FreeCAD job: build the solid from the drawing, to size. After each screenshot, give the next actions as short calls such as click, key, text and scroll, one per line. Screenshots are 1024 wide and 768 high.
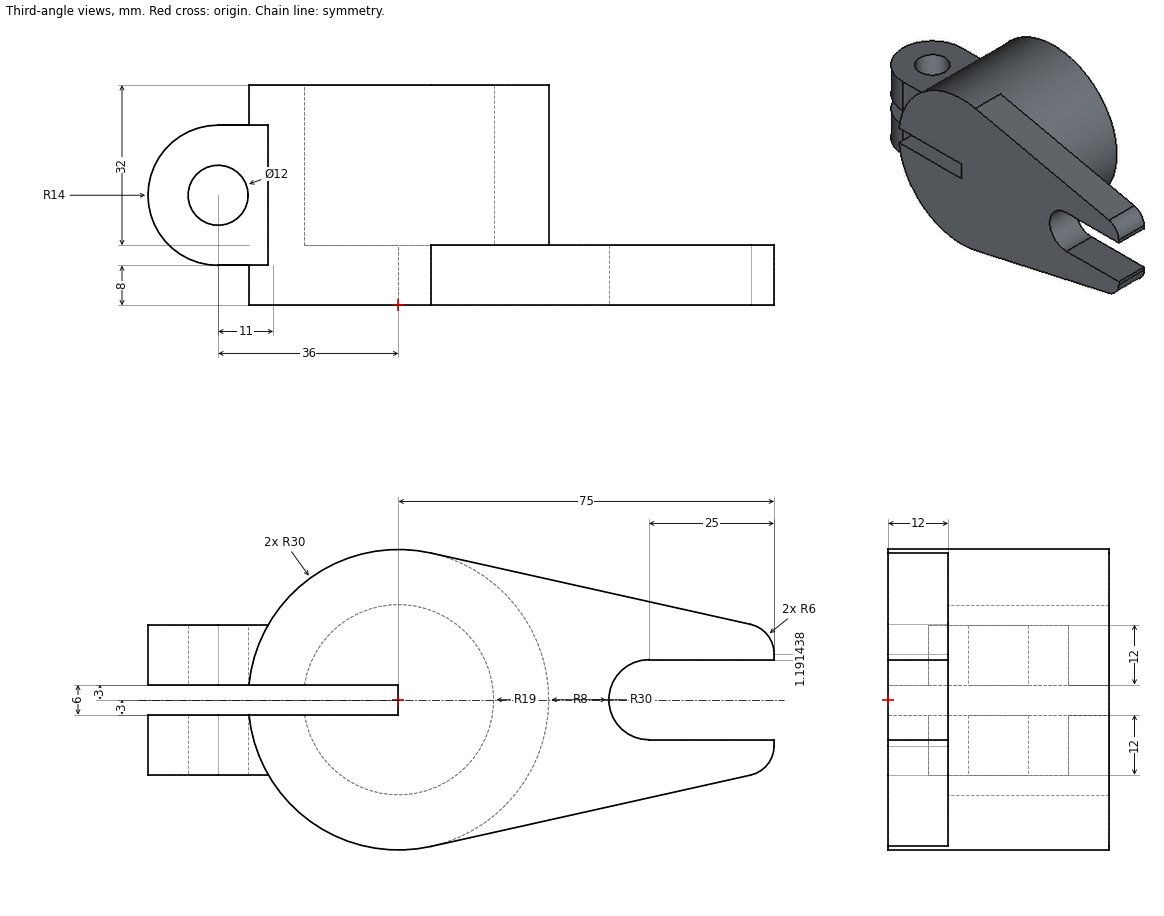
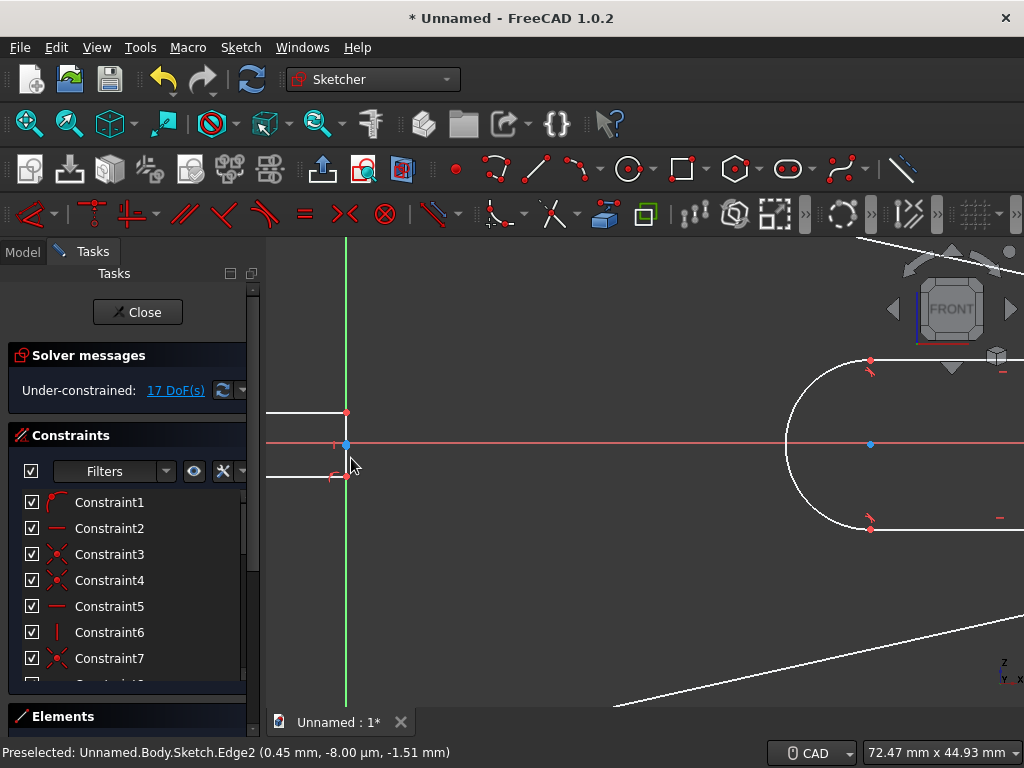
scroll(573, 489, down, 5)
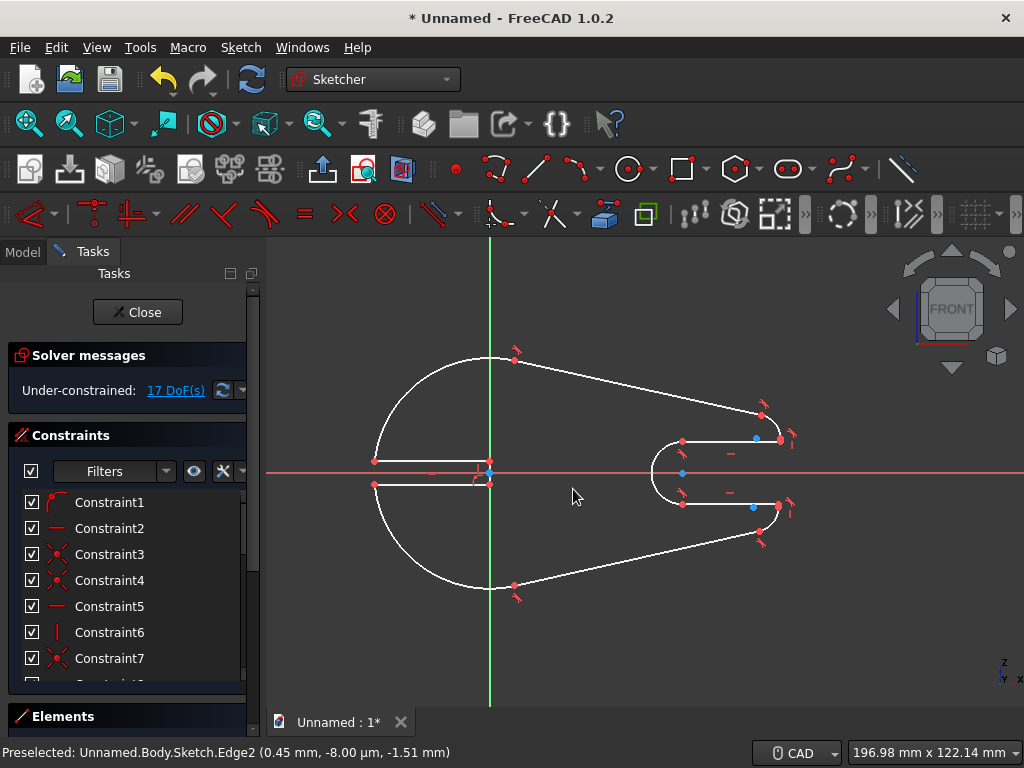
click(457, 363)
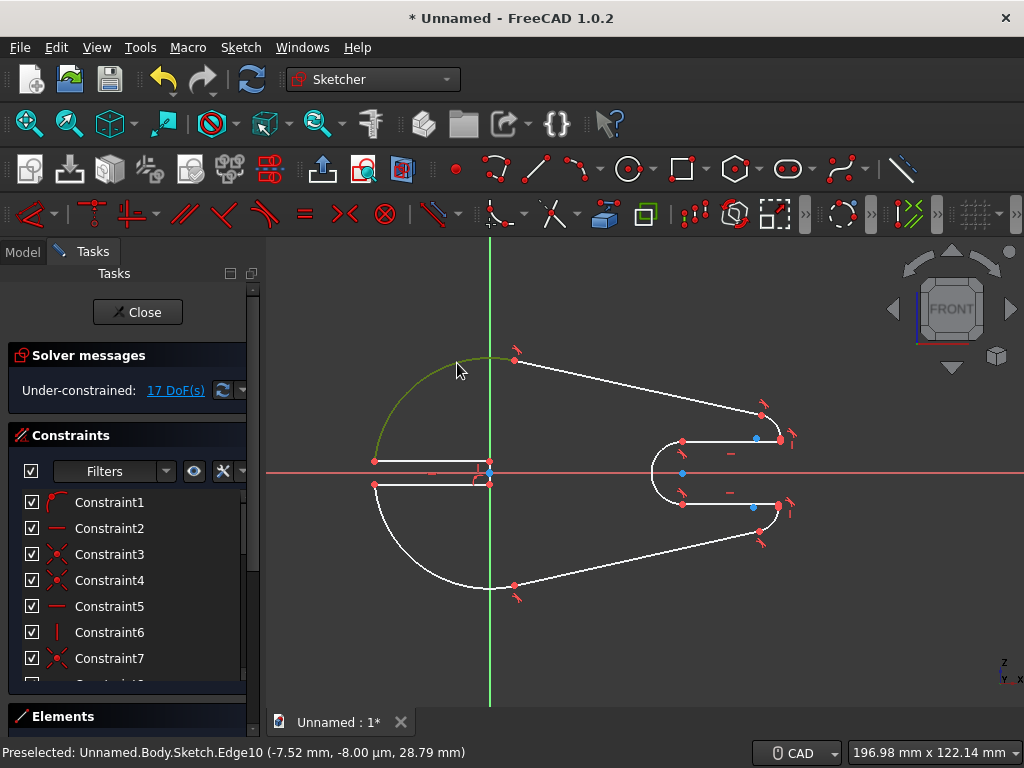
click(395, 539)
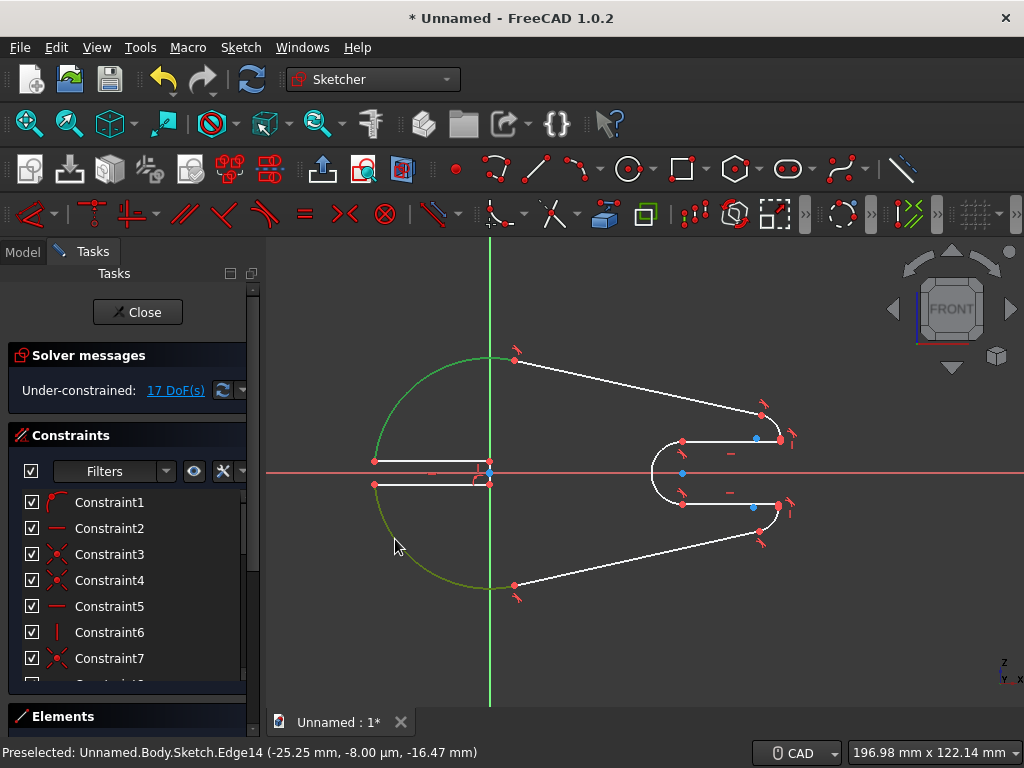
key(c)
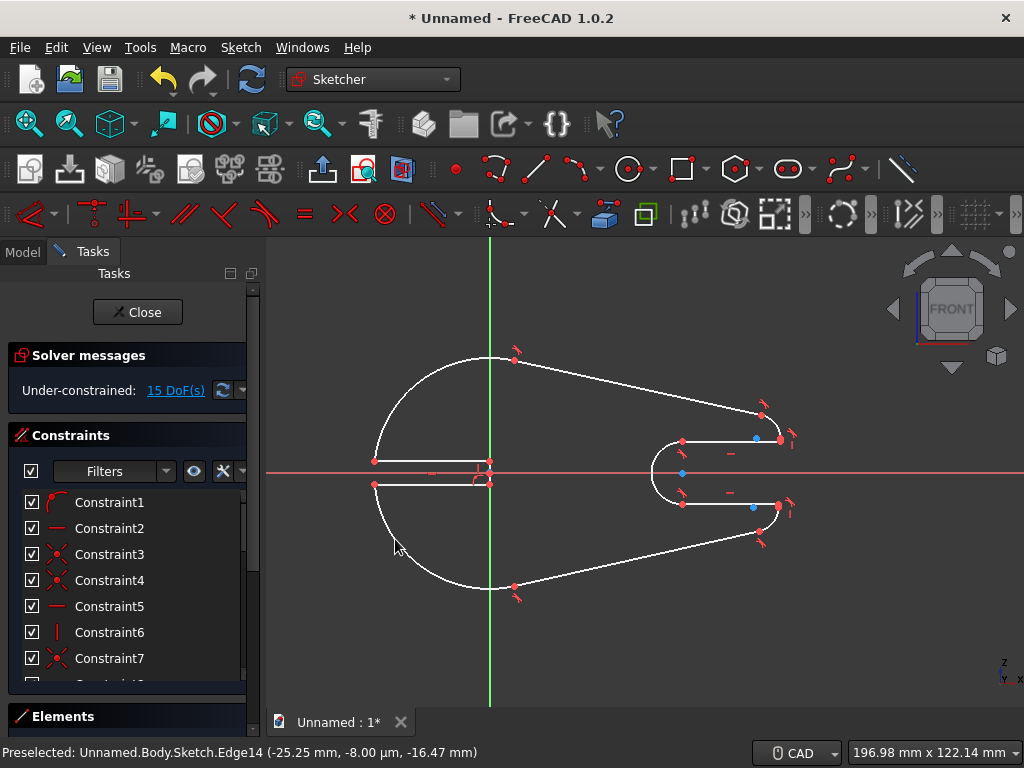
scroll(490, 473, up, 7)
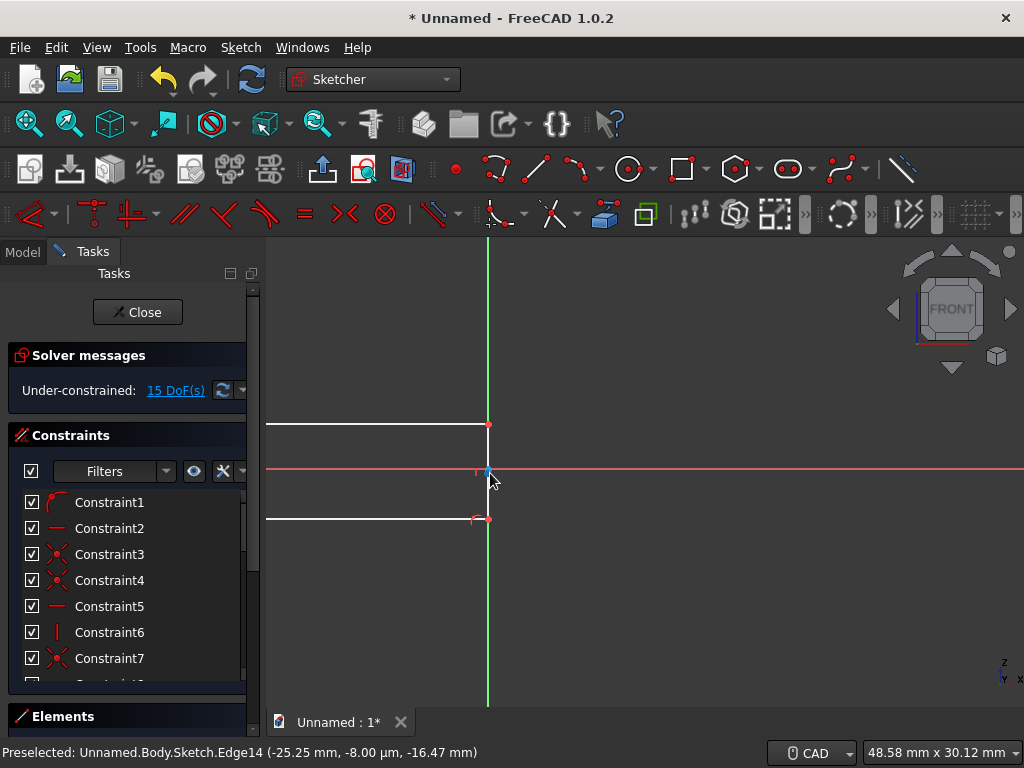
drag(478, 459, 498, 484)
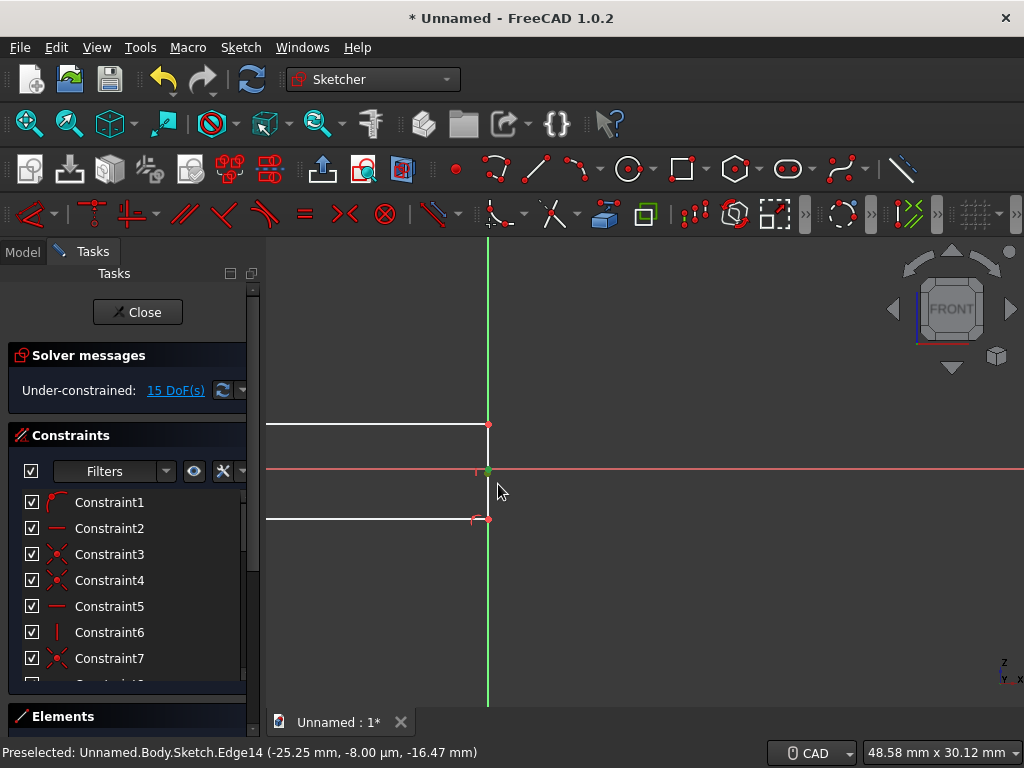
key(c)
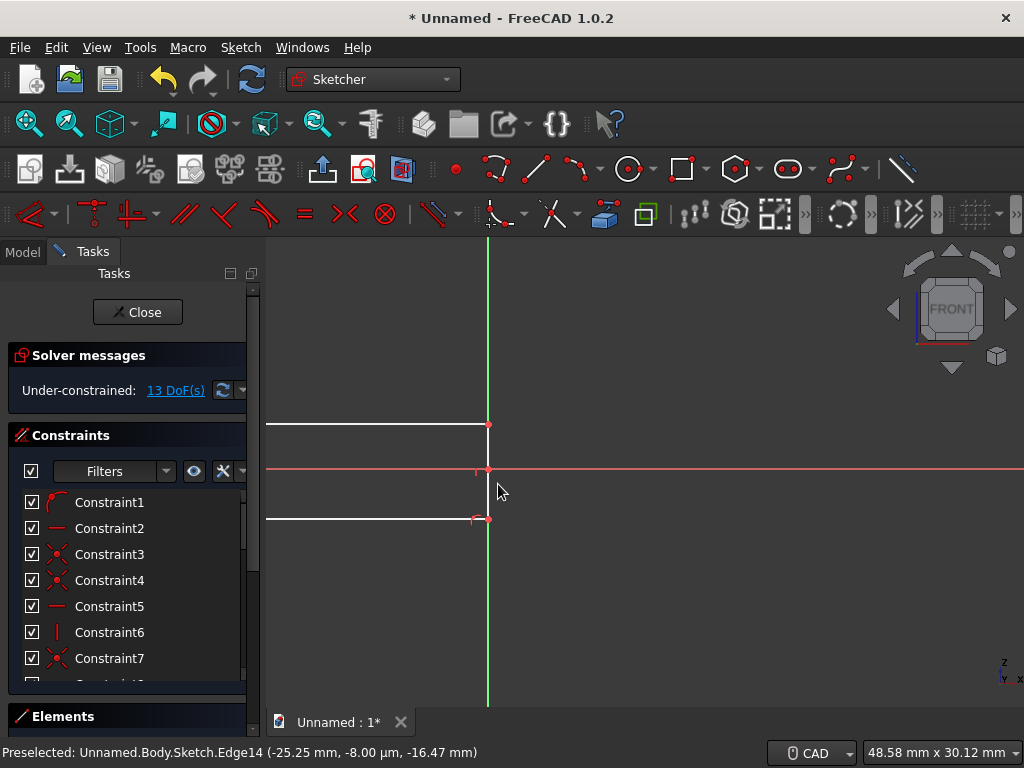
scroll(490, 473, down, 7)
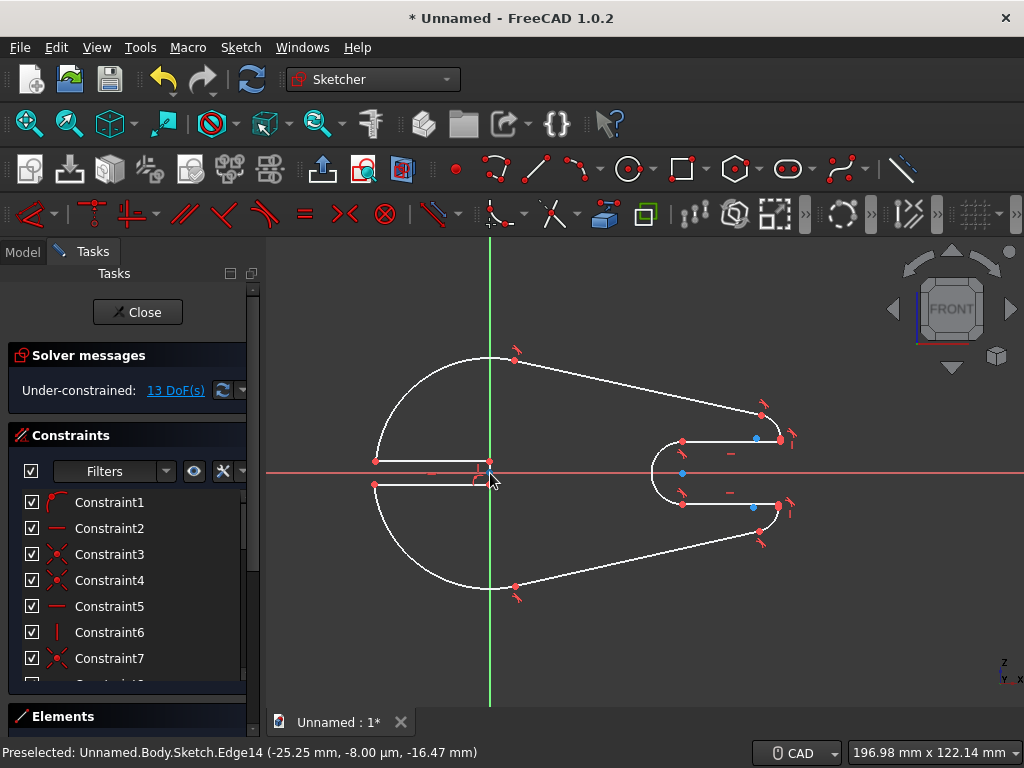
scroll(778, 429, up, 2)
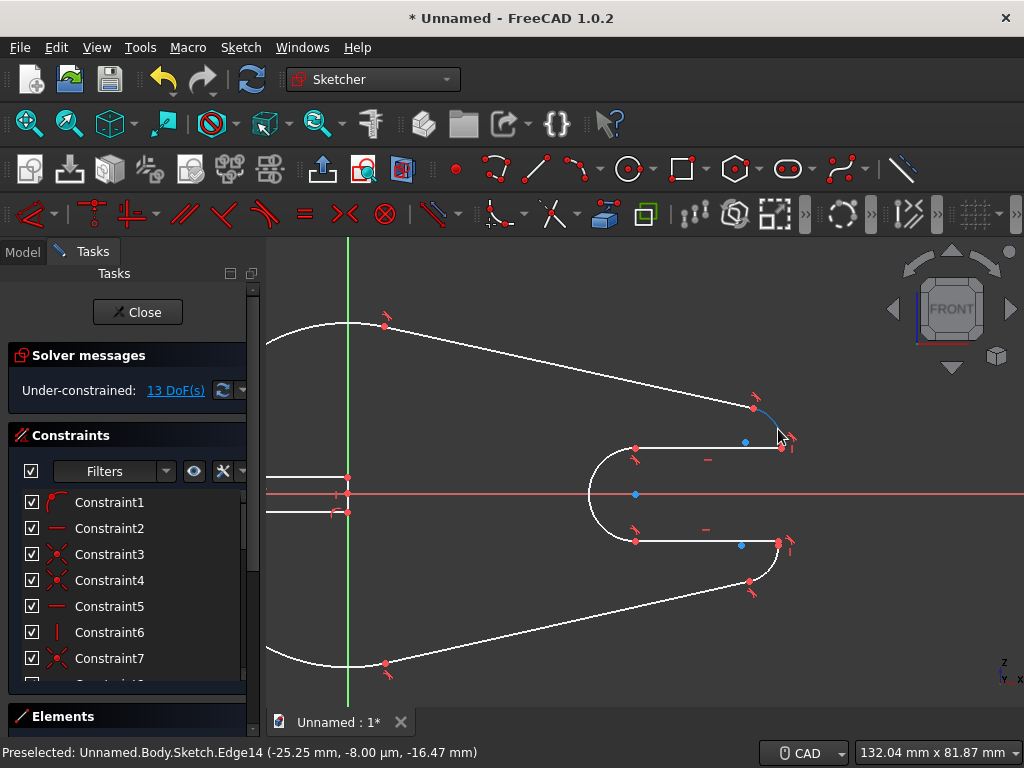
click(778, 429)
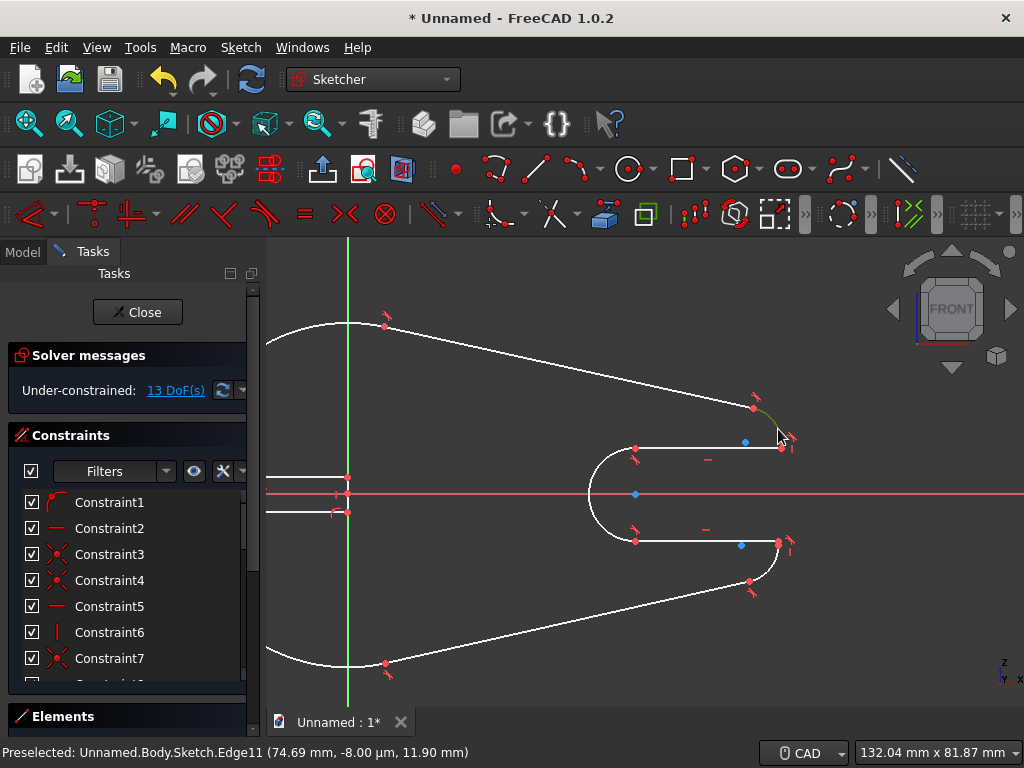
click(763, 575)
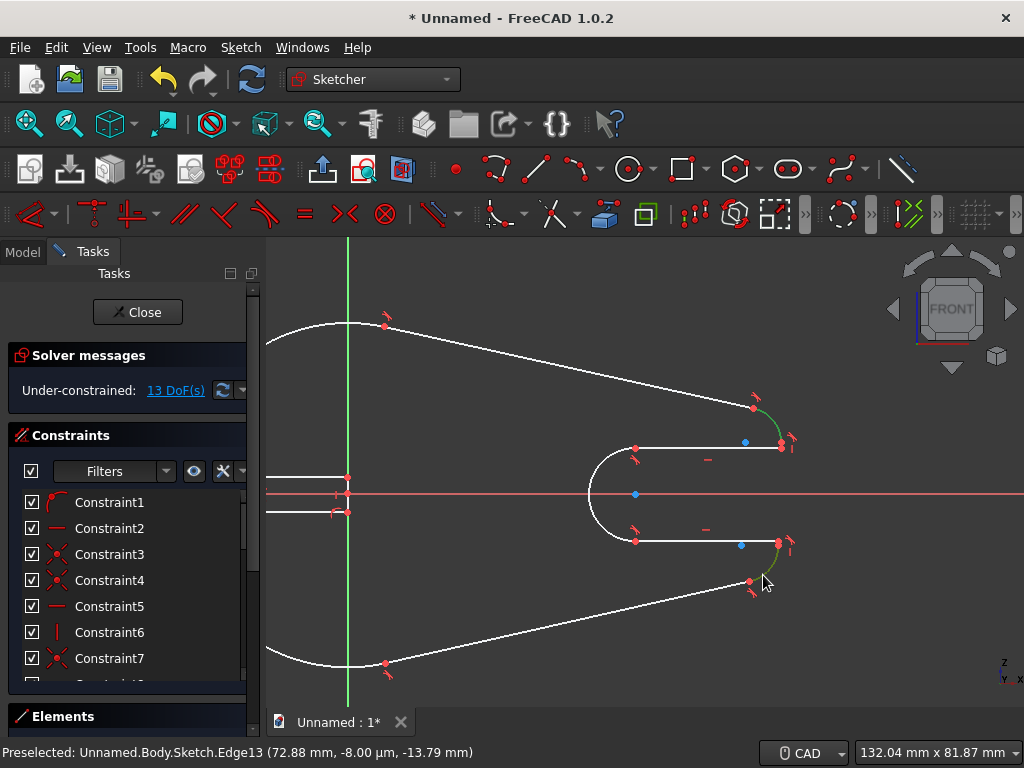
click(306, 214)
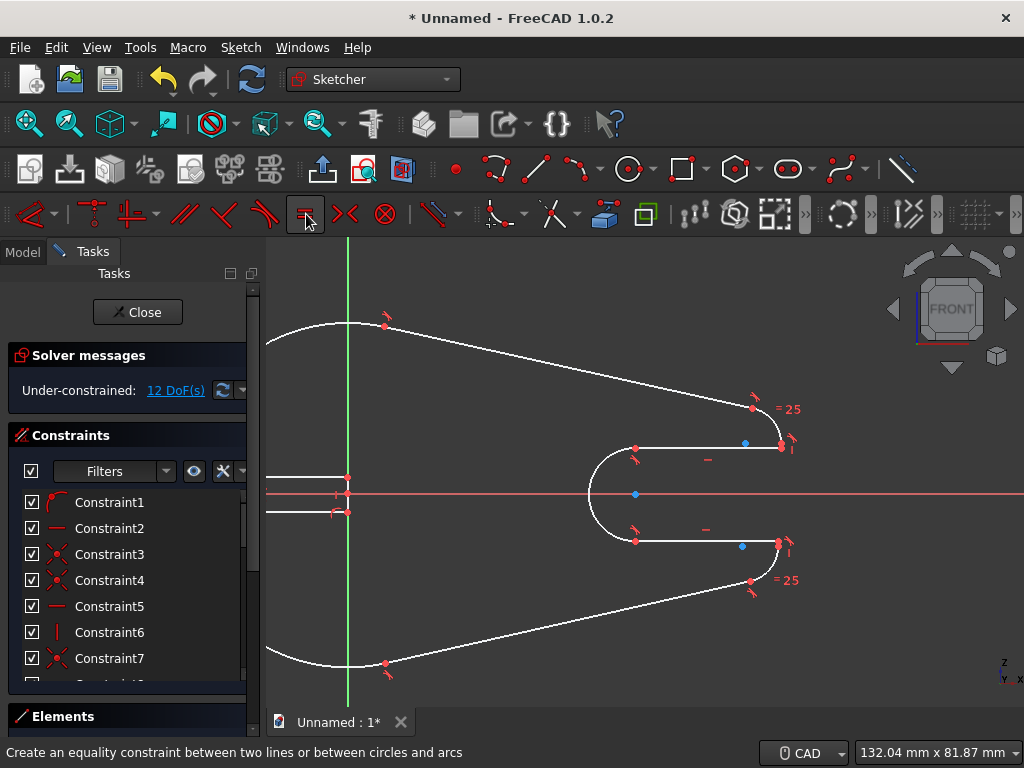
click(299, 330)